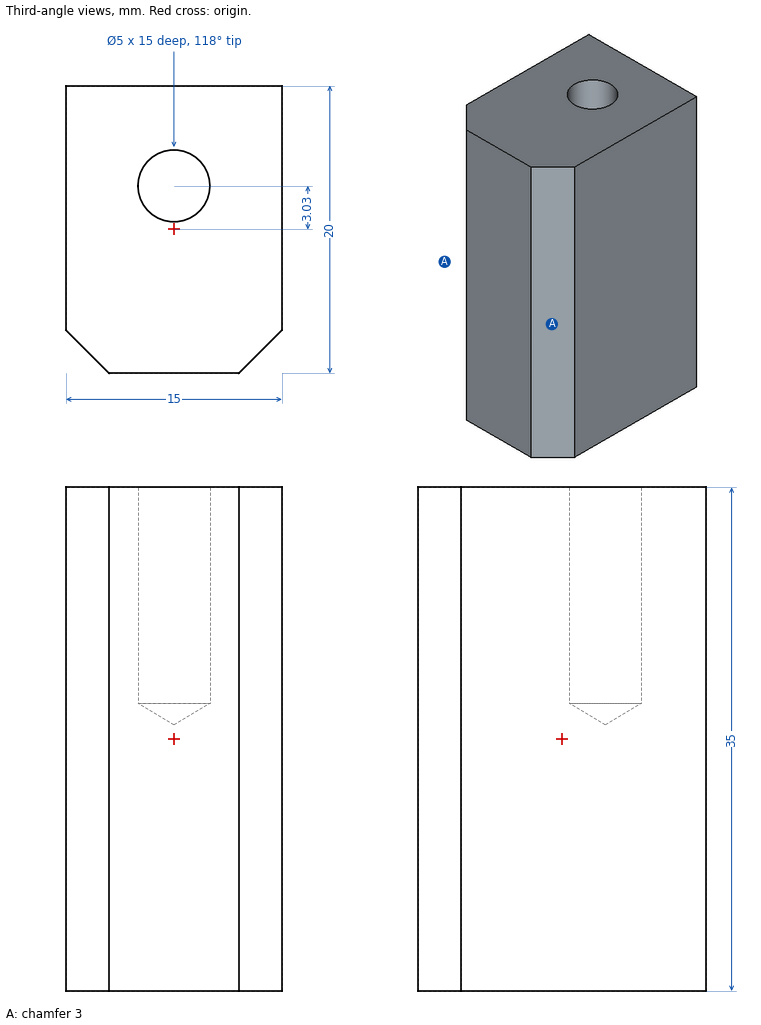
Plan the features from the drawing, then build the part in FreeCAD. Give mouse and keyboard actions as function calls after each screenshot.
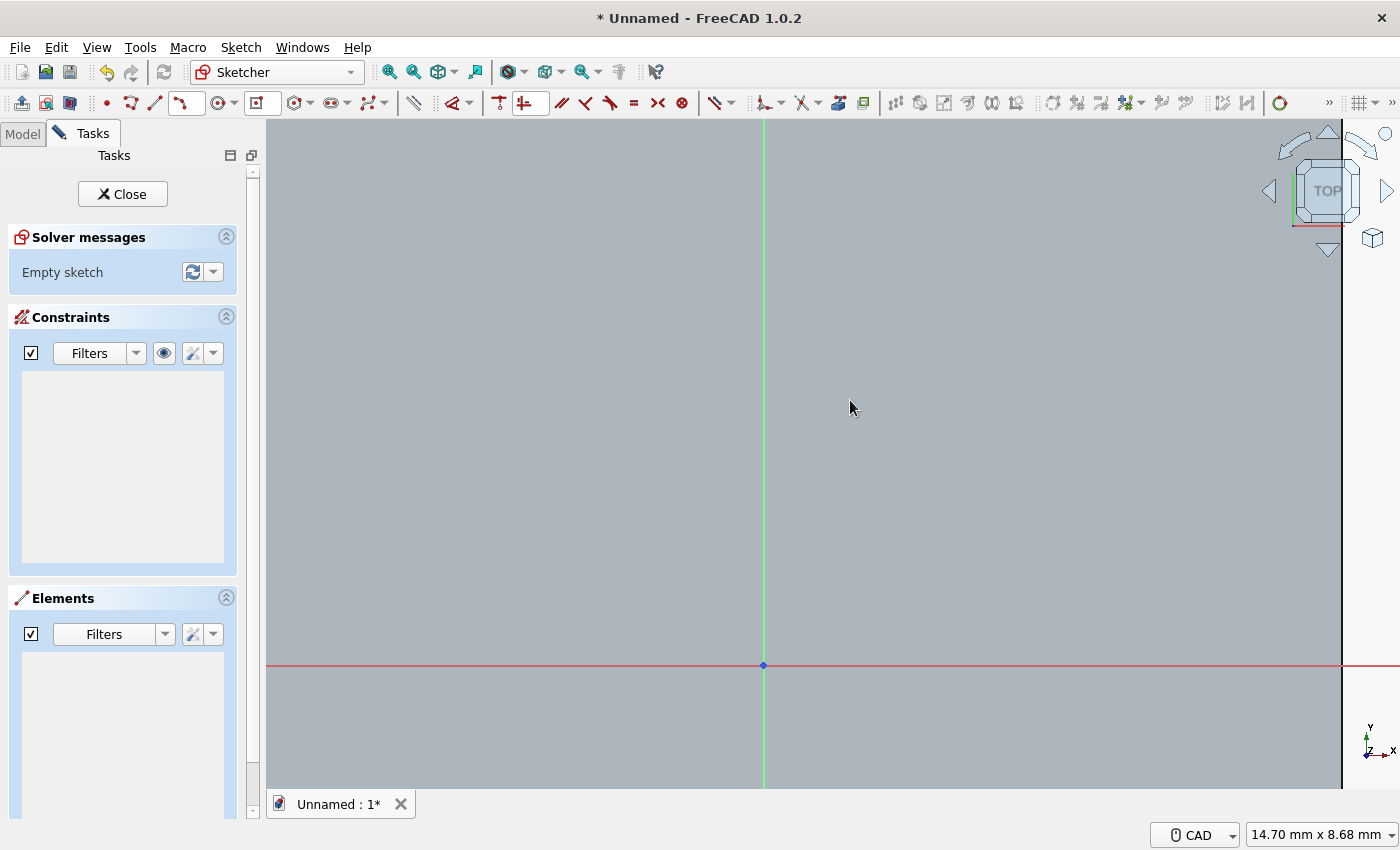
click(218, 104)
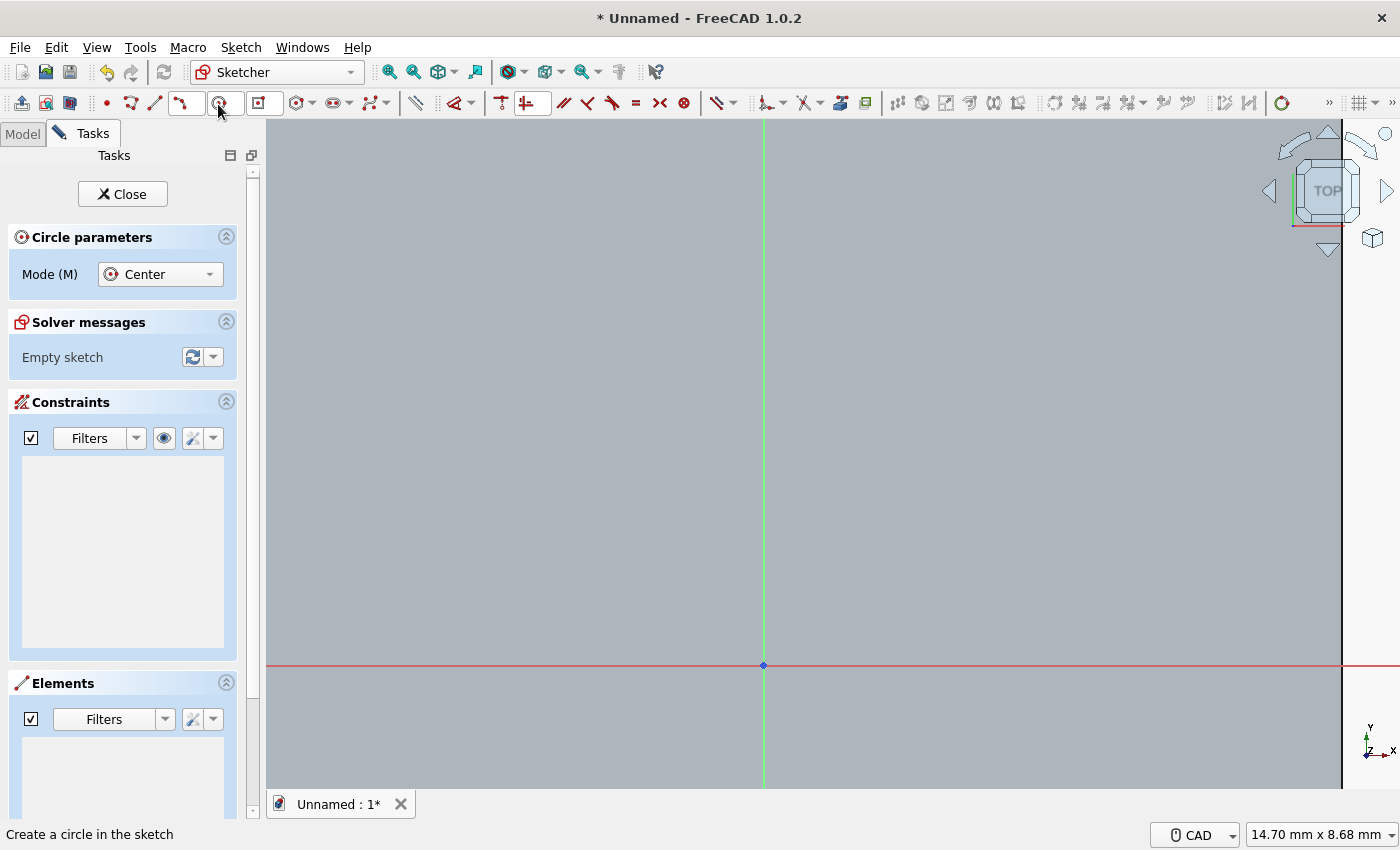
click(764, 432)
move(900, 296)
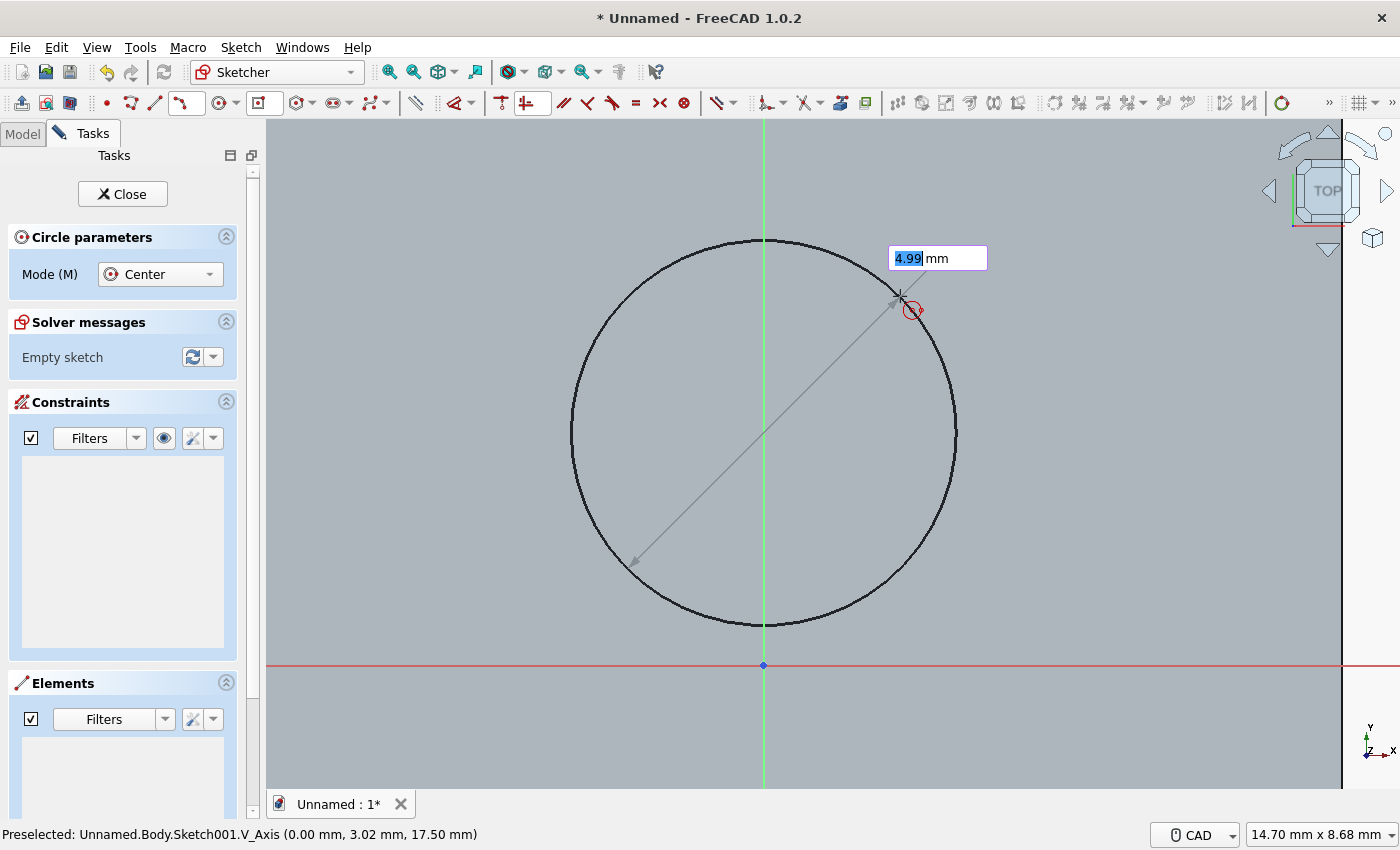
text(5)
key(Return)
key(Escape)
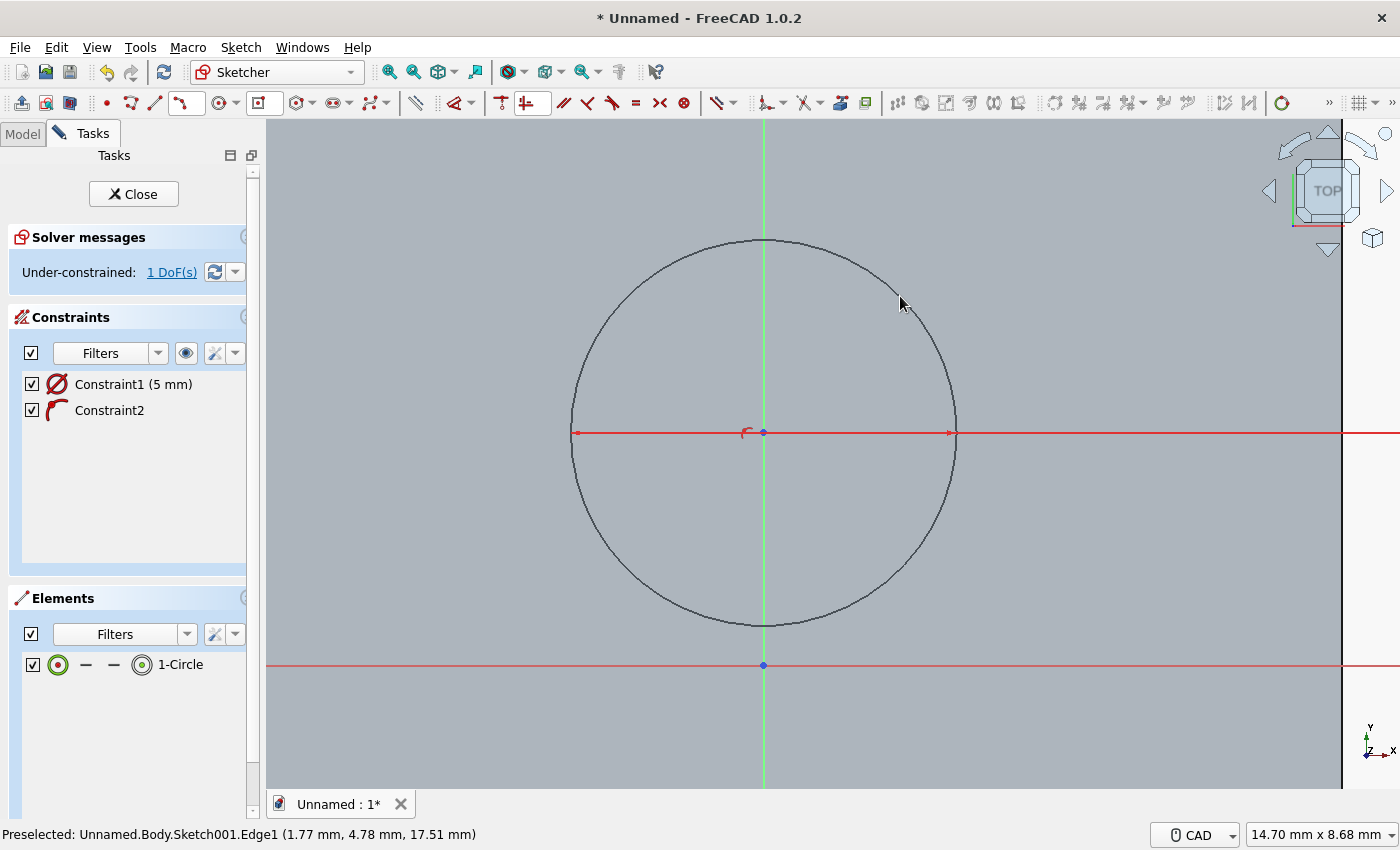
click(454, 104)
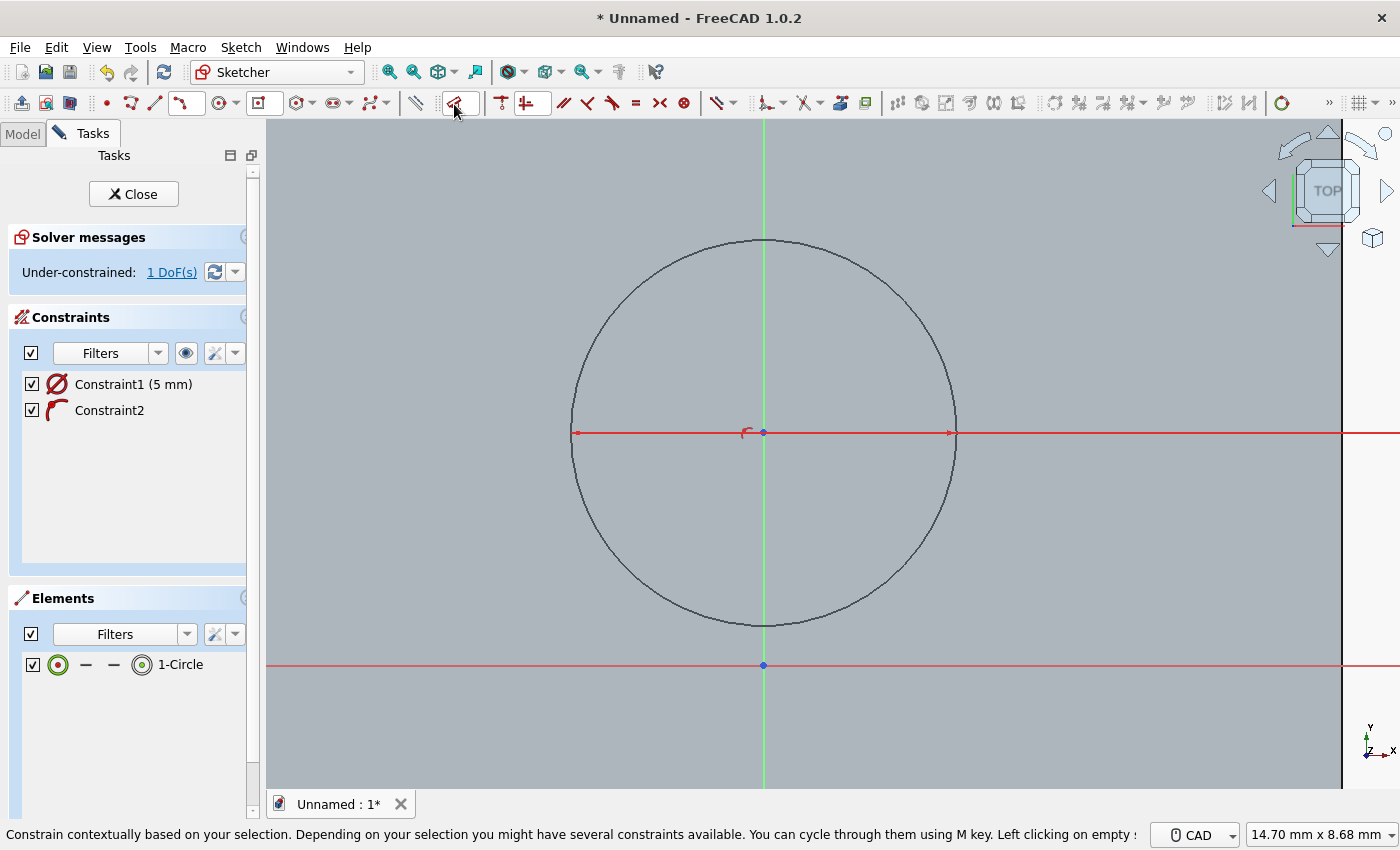
click(764, 433)
click(798, 549)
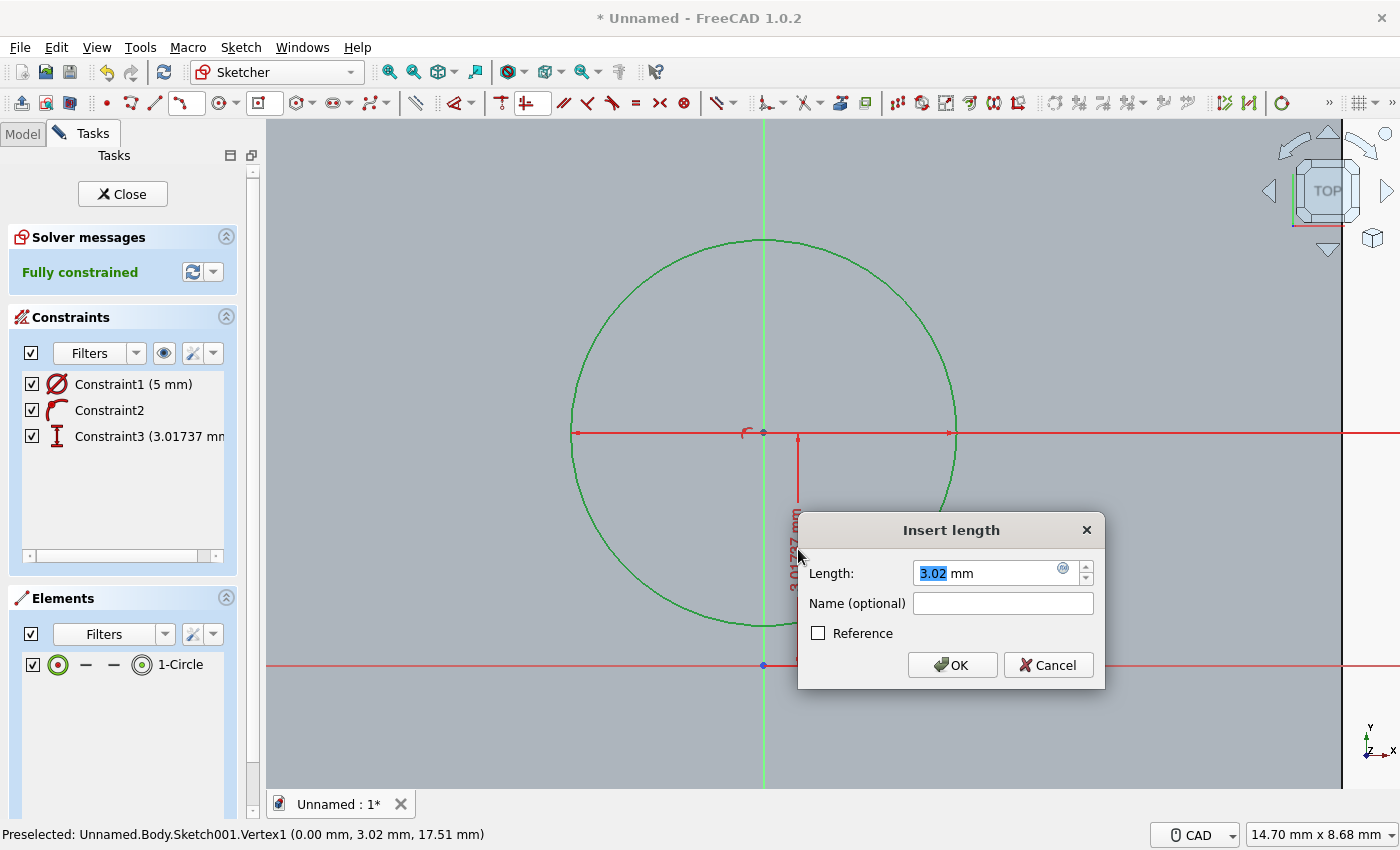
text(3.03)
key(Return)
key(Escape)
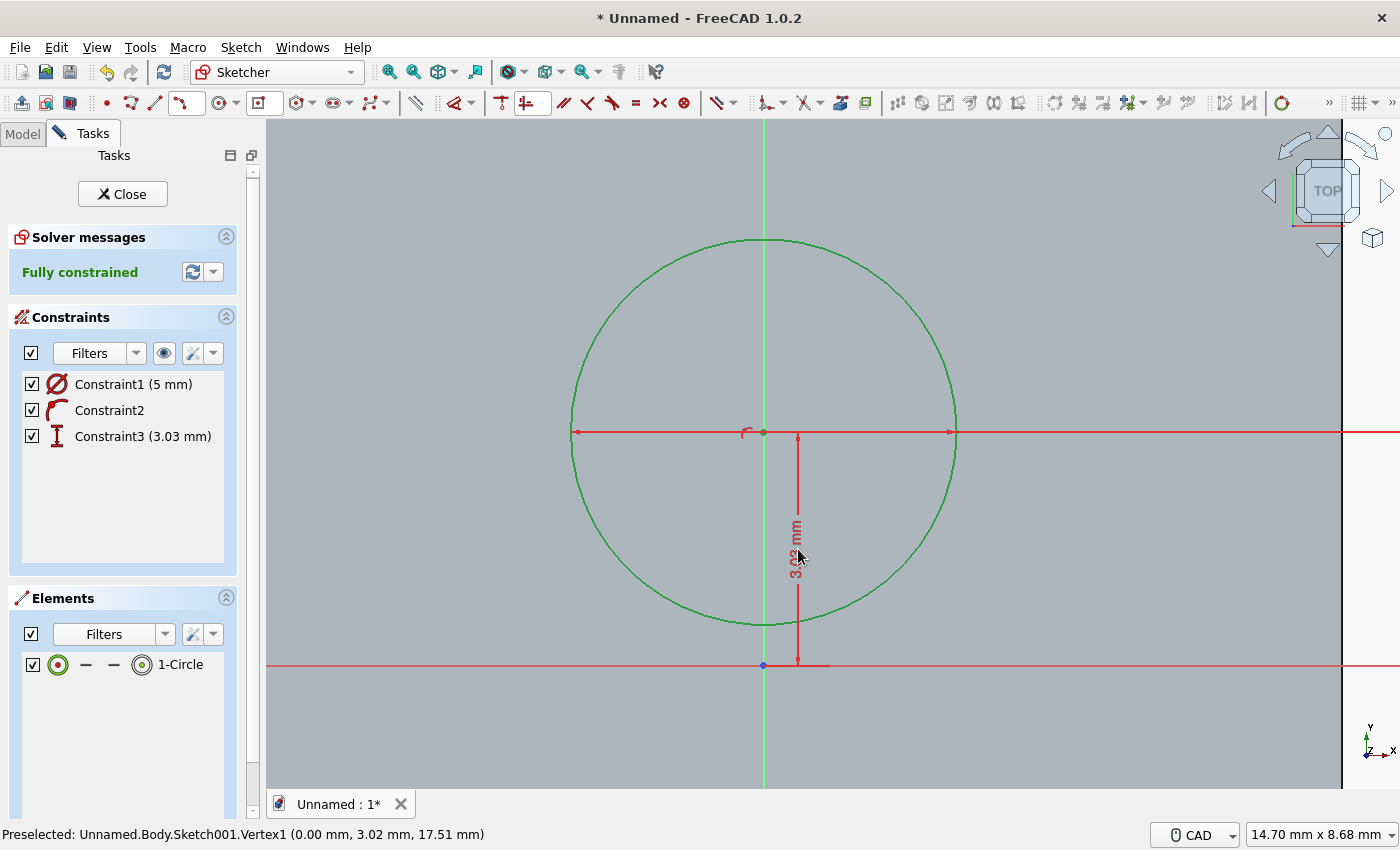
click(123, 194)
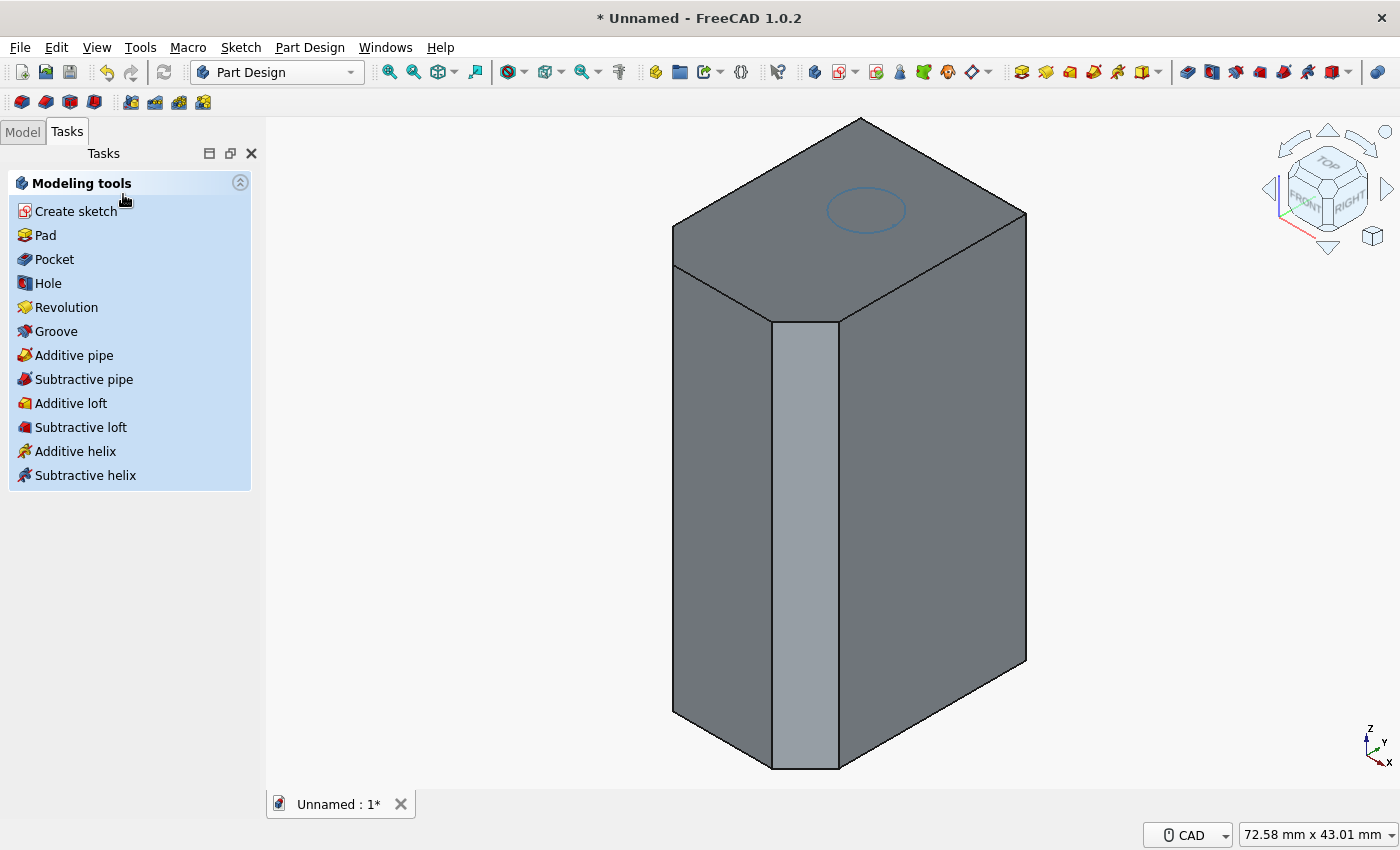
click(1212, 72)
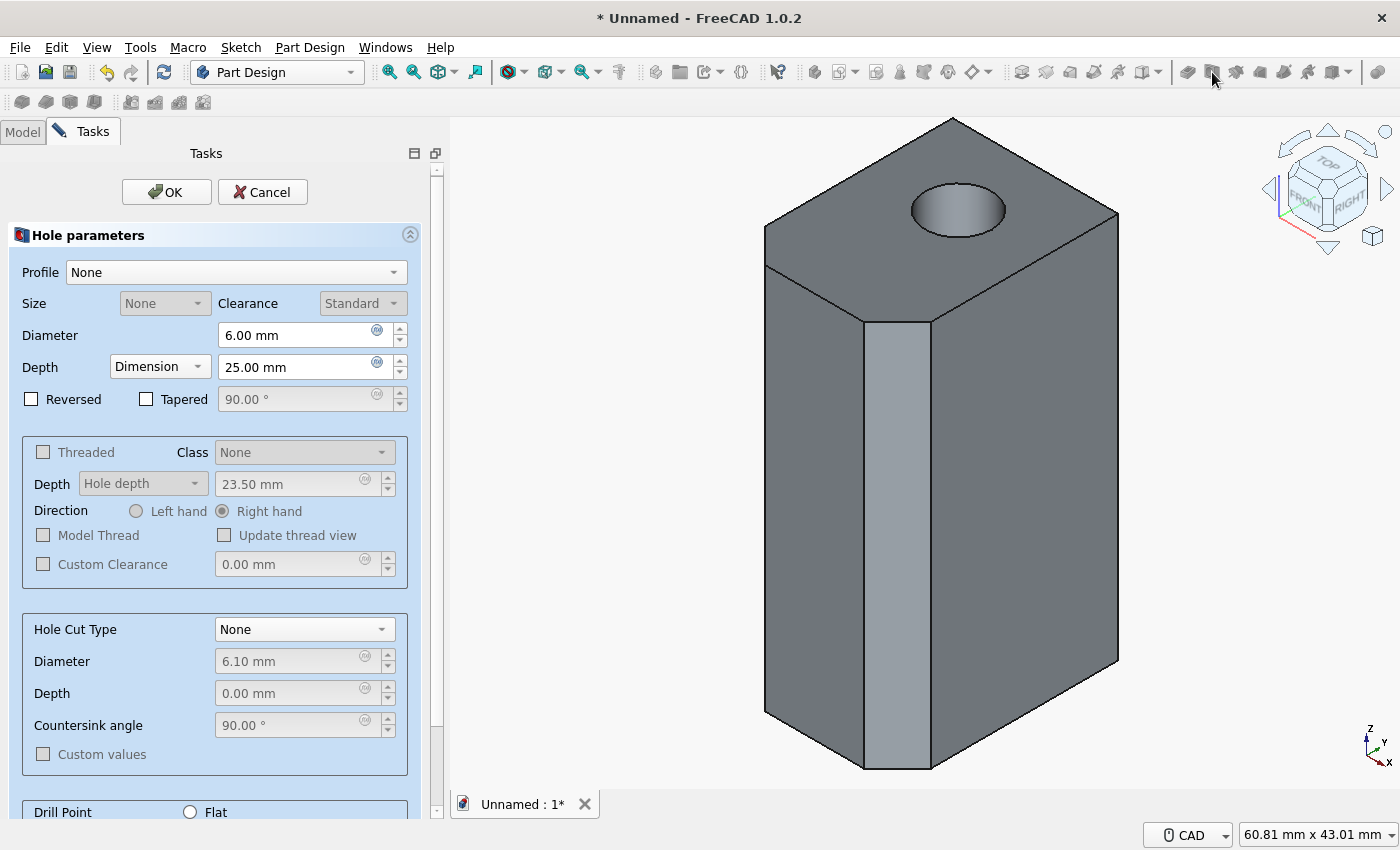
triple_click(305, 335)